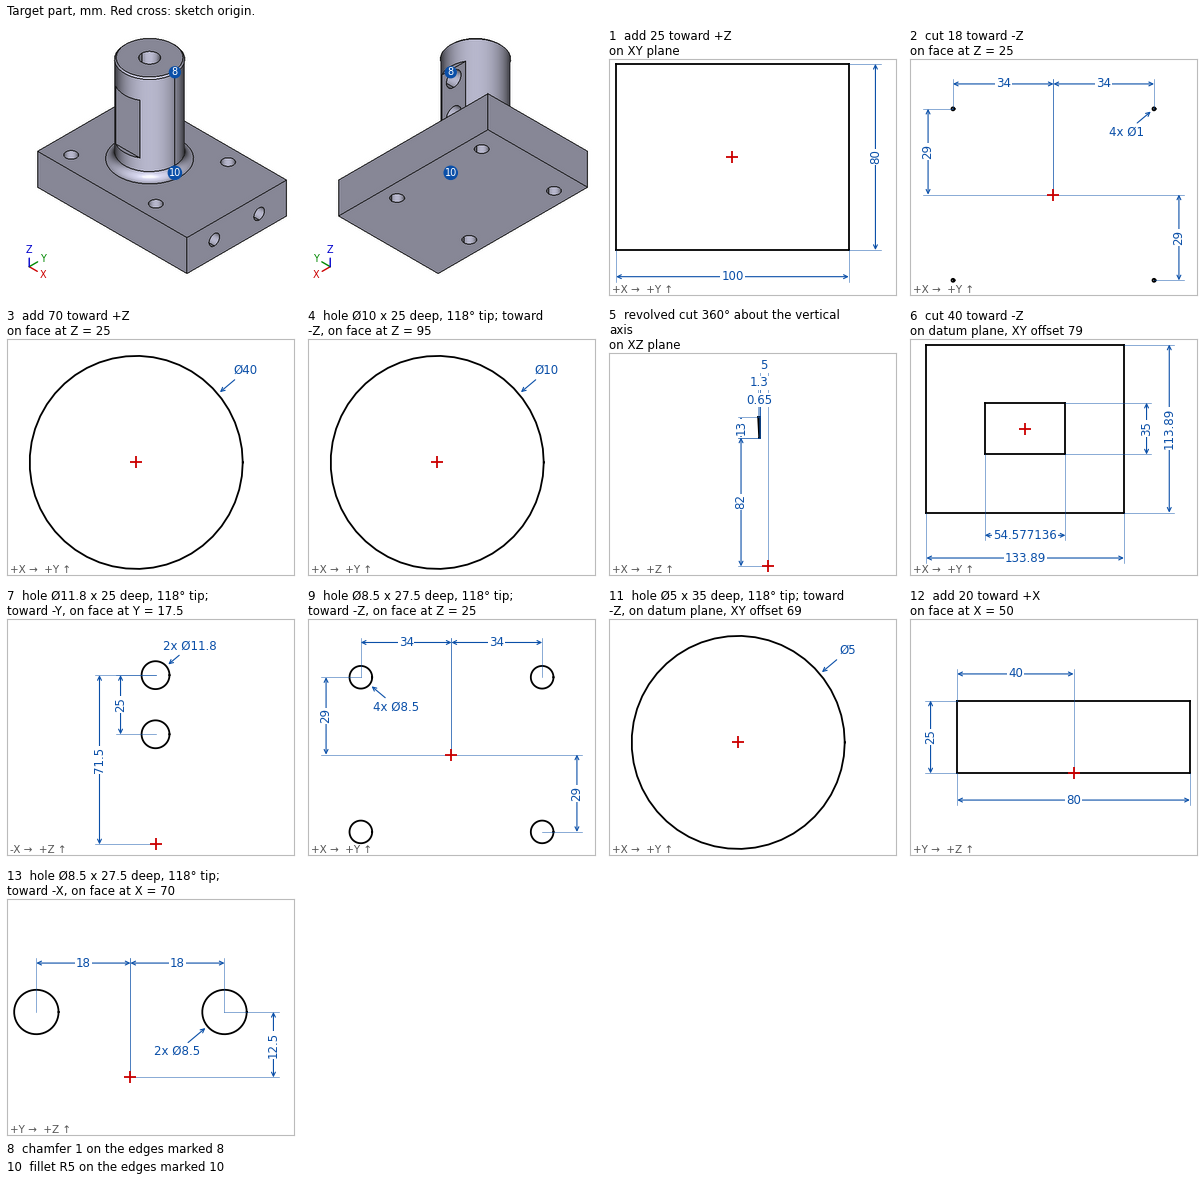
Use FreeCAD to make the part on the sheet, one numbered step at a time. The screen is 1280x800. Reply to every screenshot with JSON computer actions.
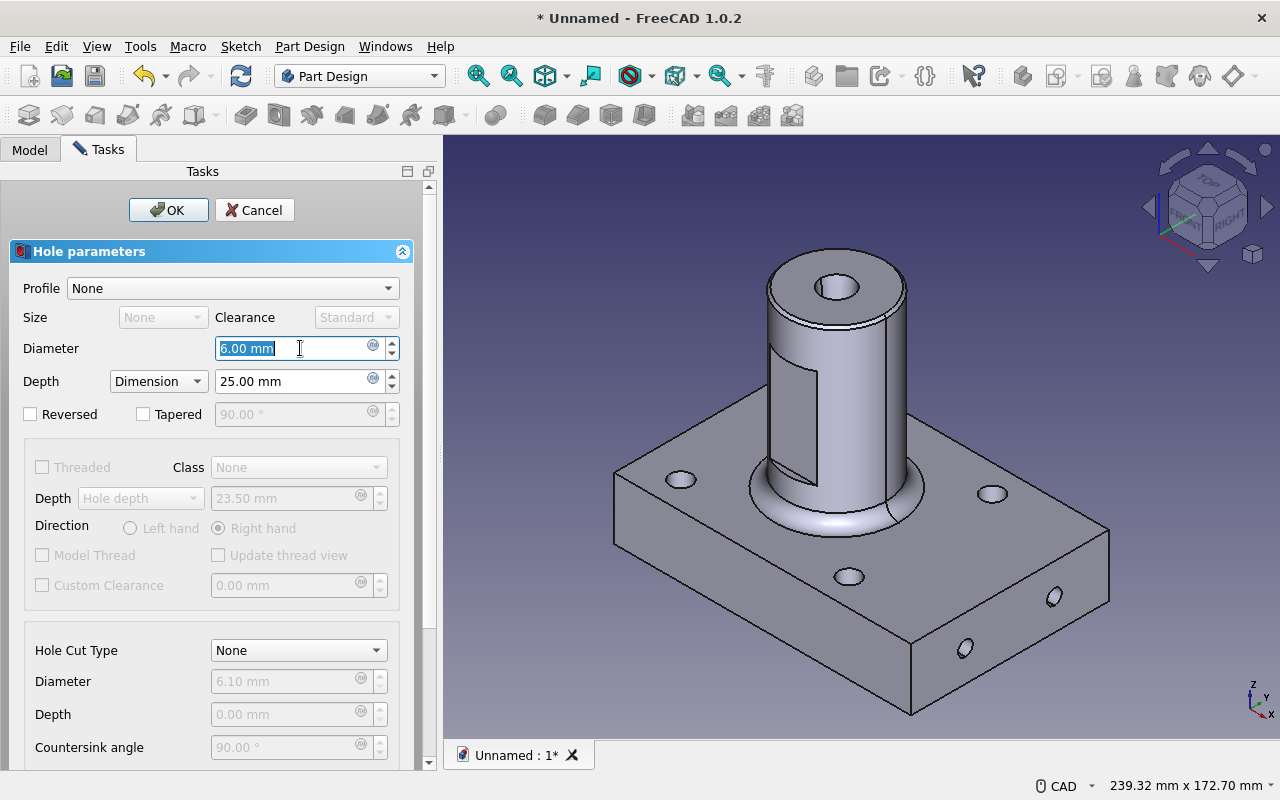
{"action": "type", "text": "8.5"}
{"action": "key", "text": "Tab"}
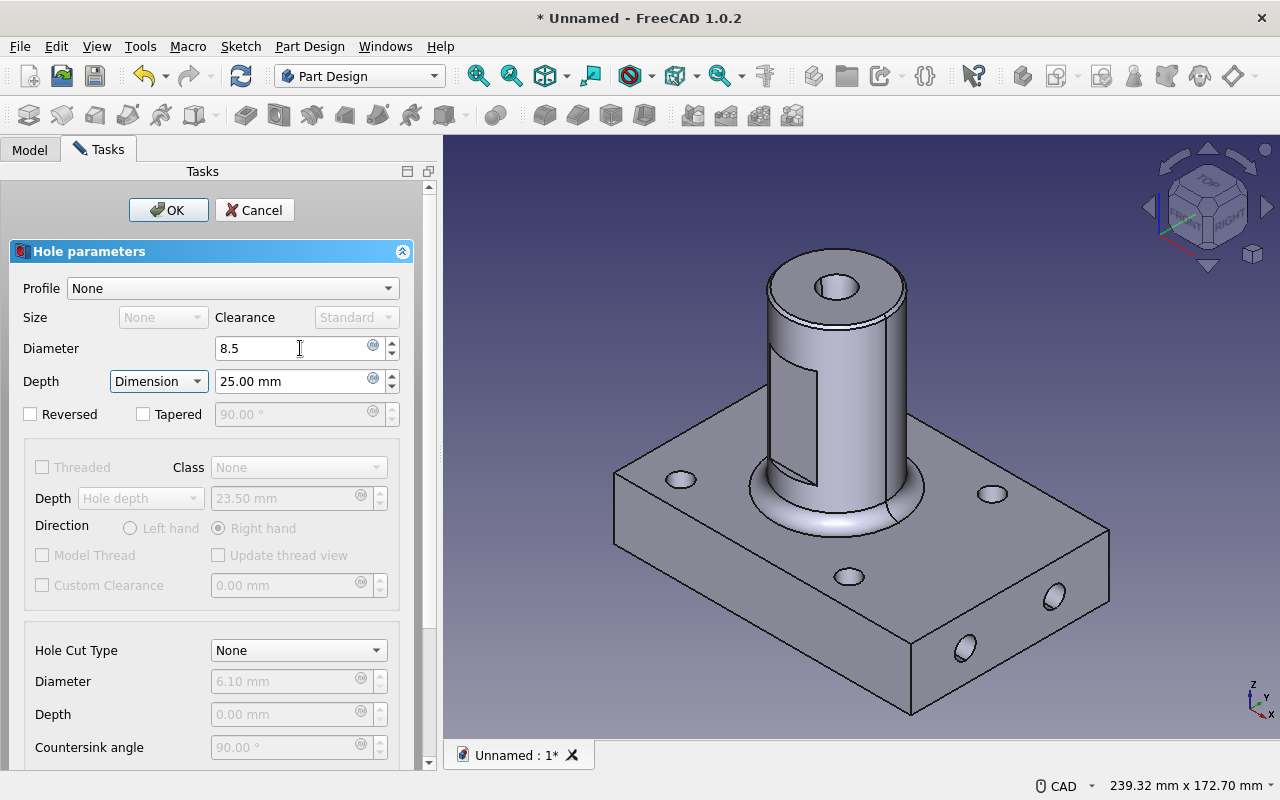
{"action": "triple_click", "coordinate": [300, 382]}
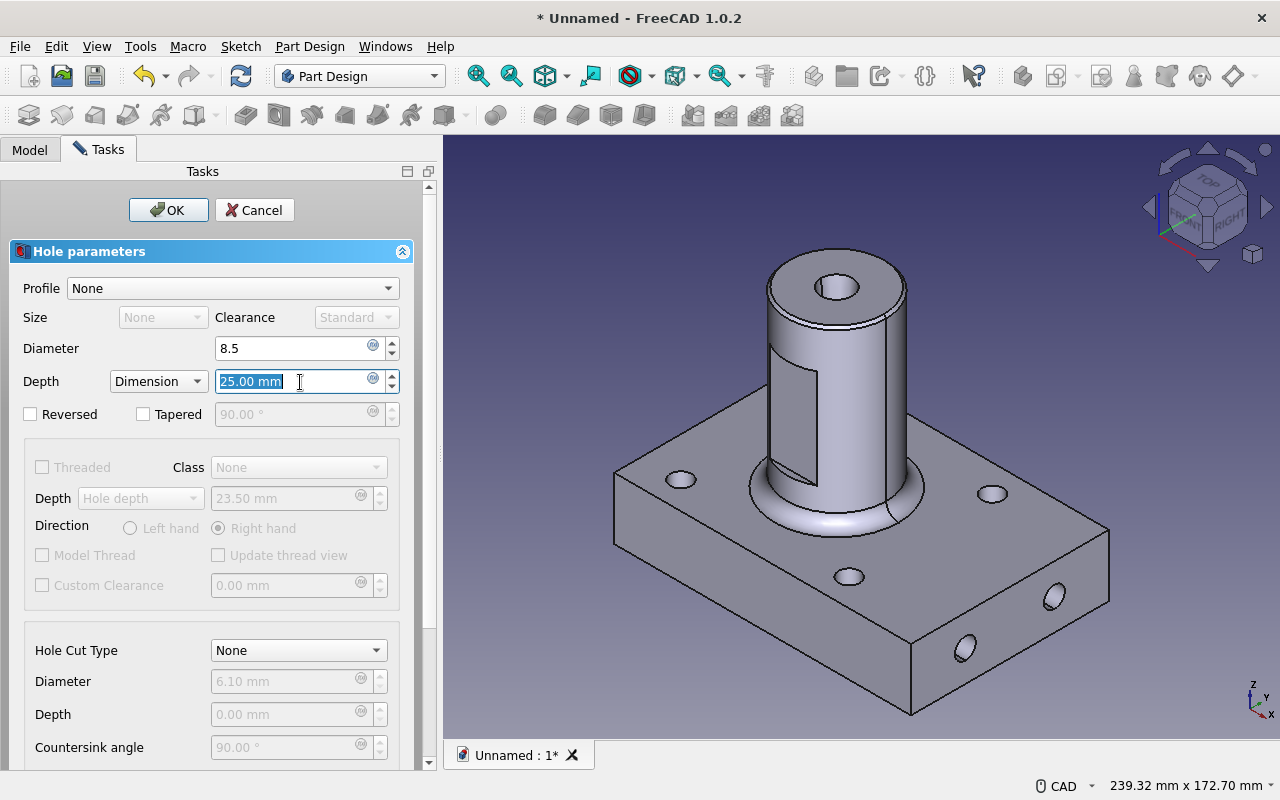
{"action": "type", "text": "27.5"}
{"action": "key", "text": "Tab"}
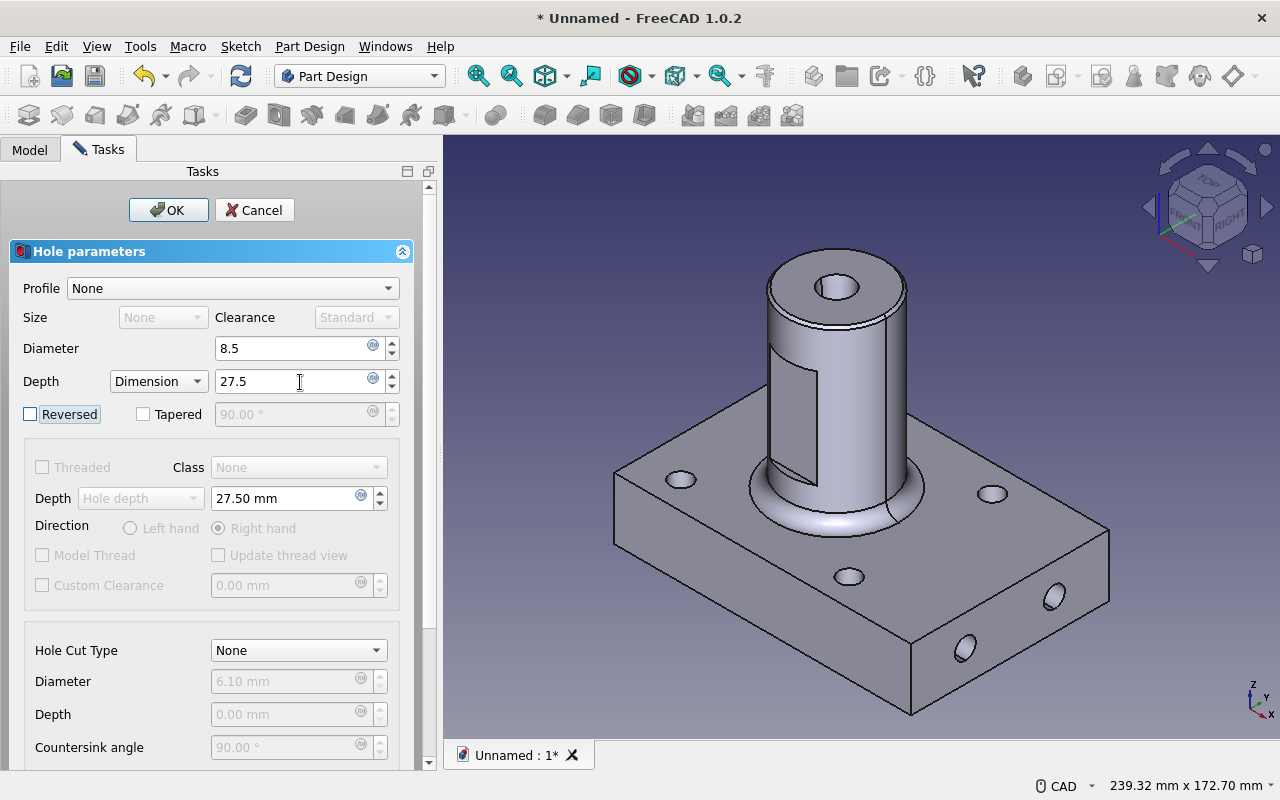
{"action": "left_click", "coordinate": [169, 210]}